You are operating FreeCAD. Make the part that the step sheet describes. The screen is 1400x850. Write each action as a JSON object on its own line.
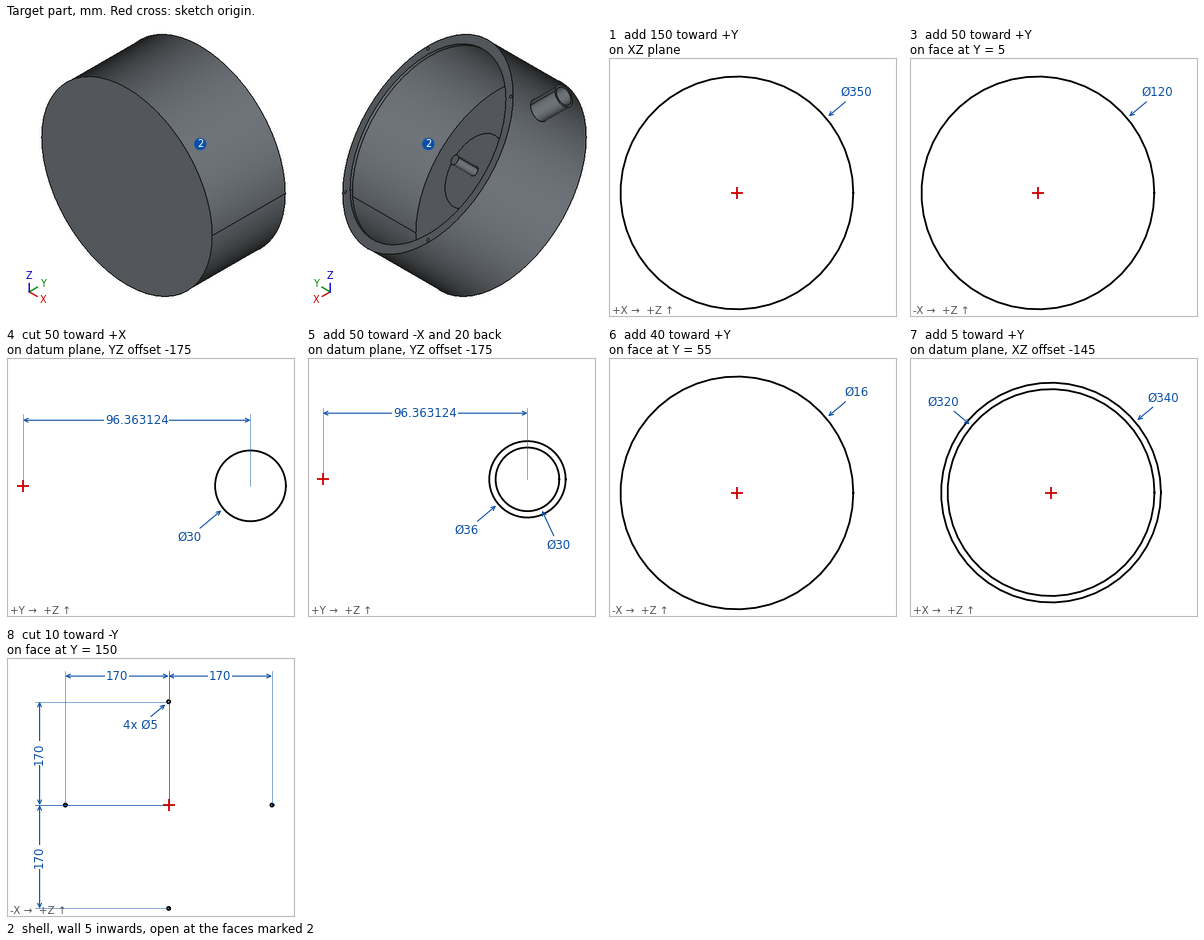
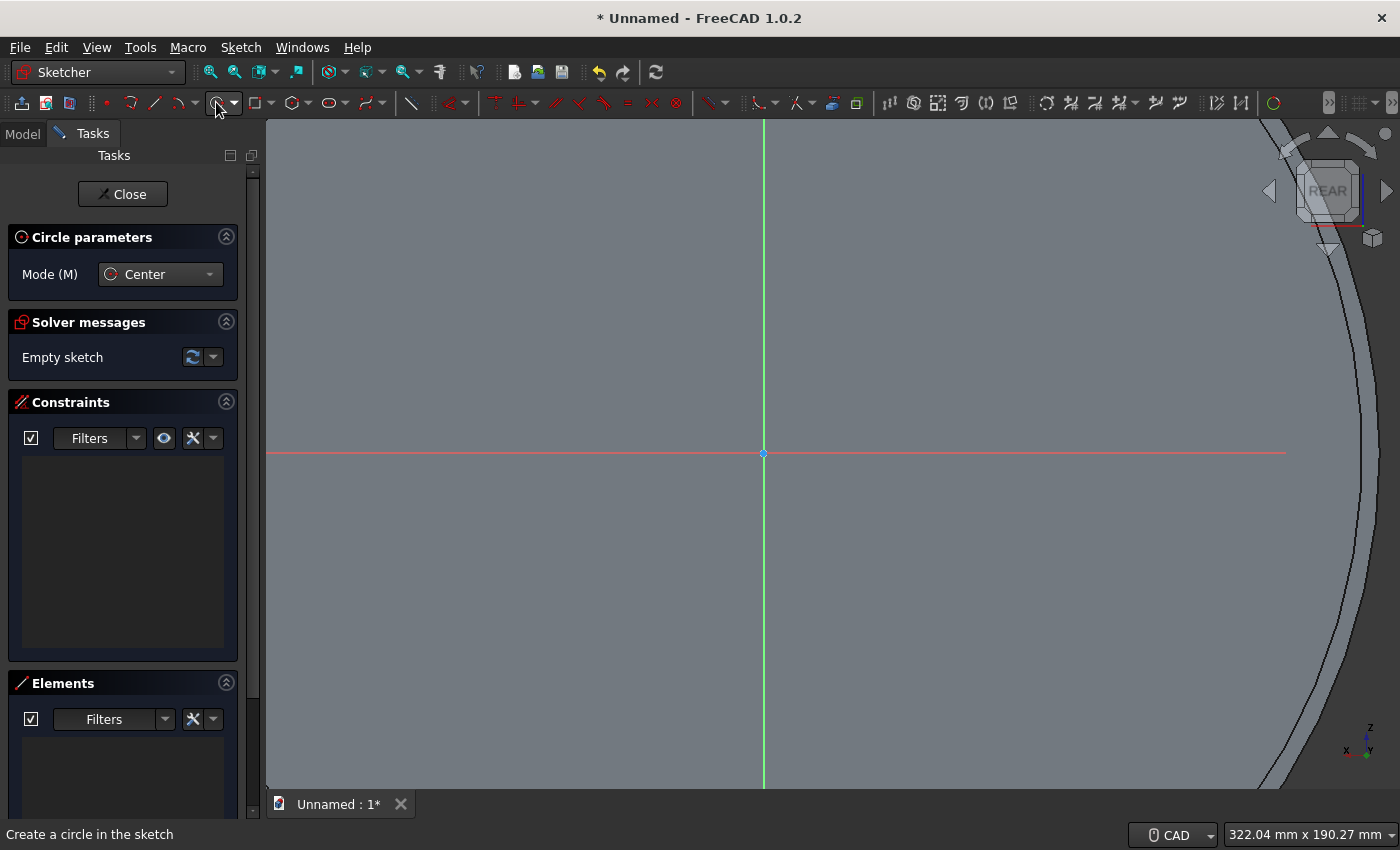
{"action": "left_click", "coordinate": [764, 453]}
{"action": "mouse_move", "coordinate": [913, 304]}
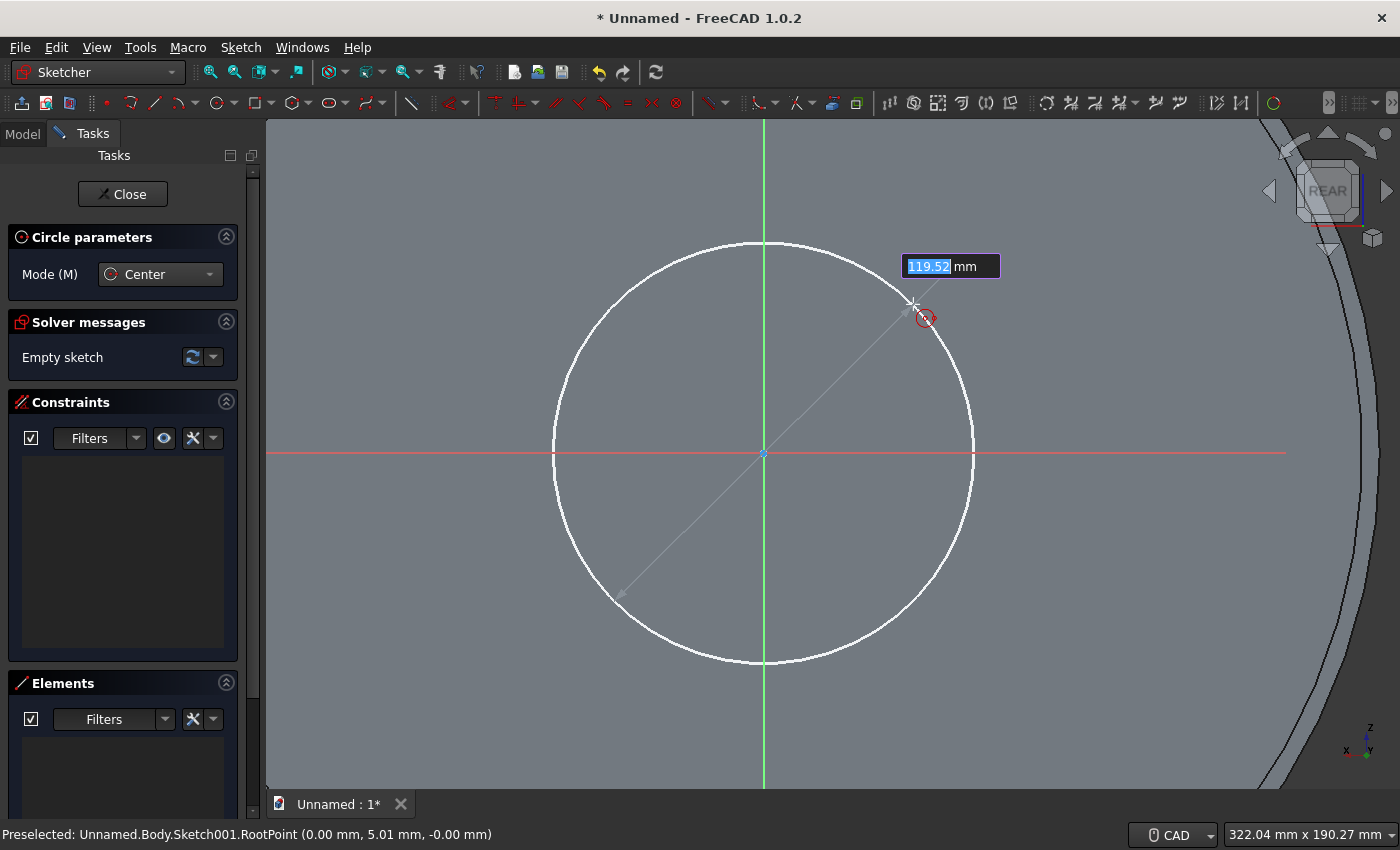
{"action": "type", "text": "120"}
{"action": "key", "text": "Return"}
{"action": "key", "text": "Escape"}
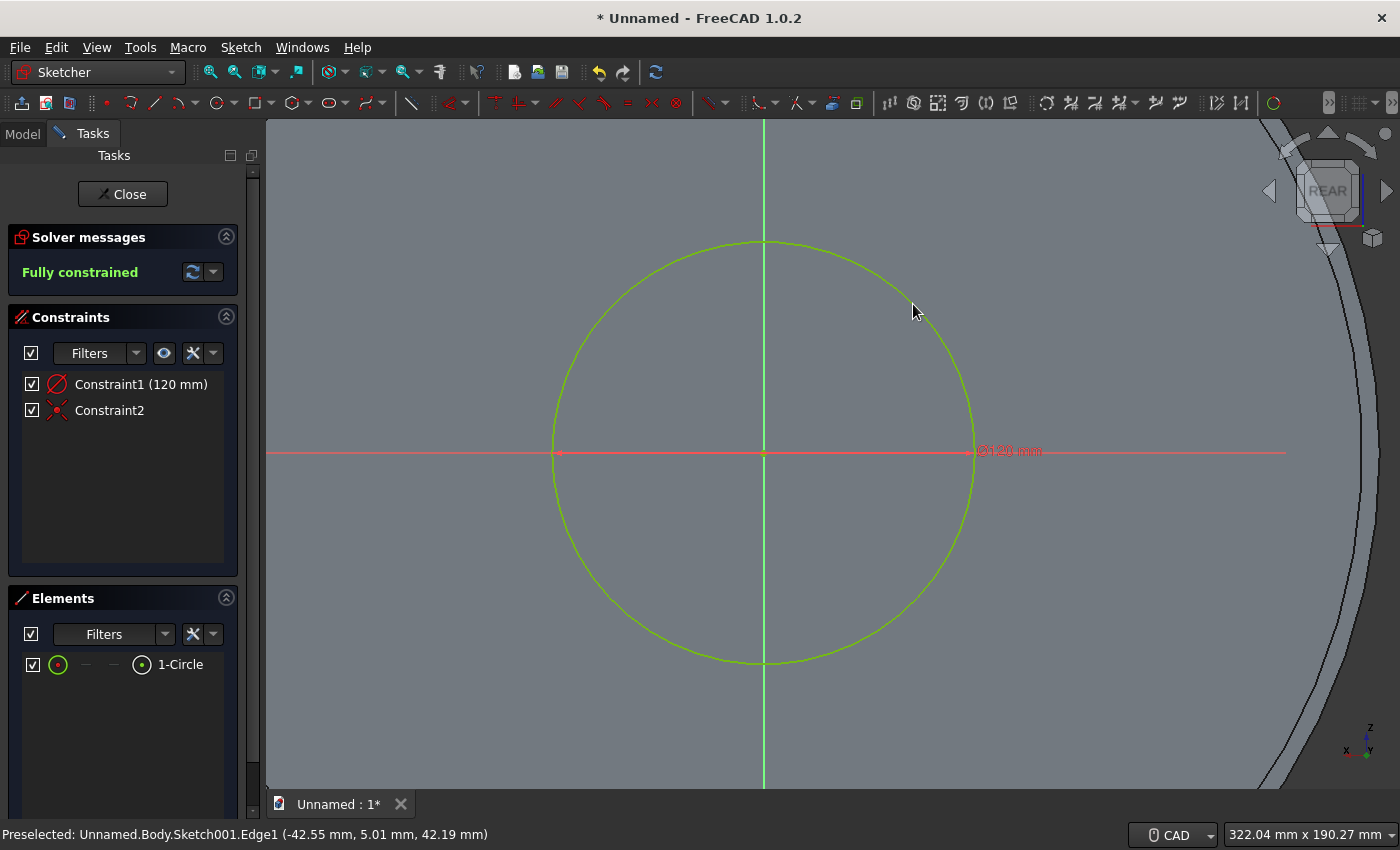
{"action": "left_click", "coordinate": [123, 194]}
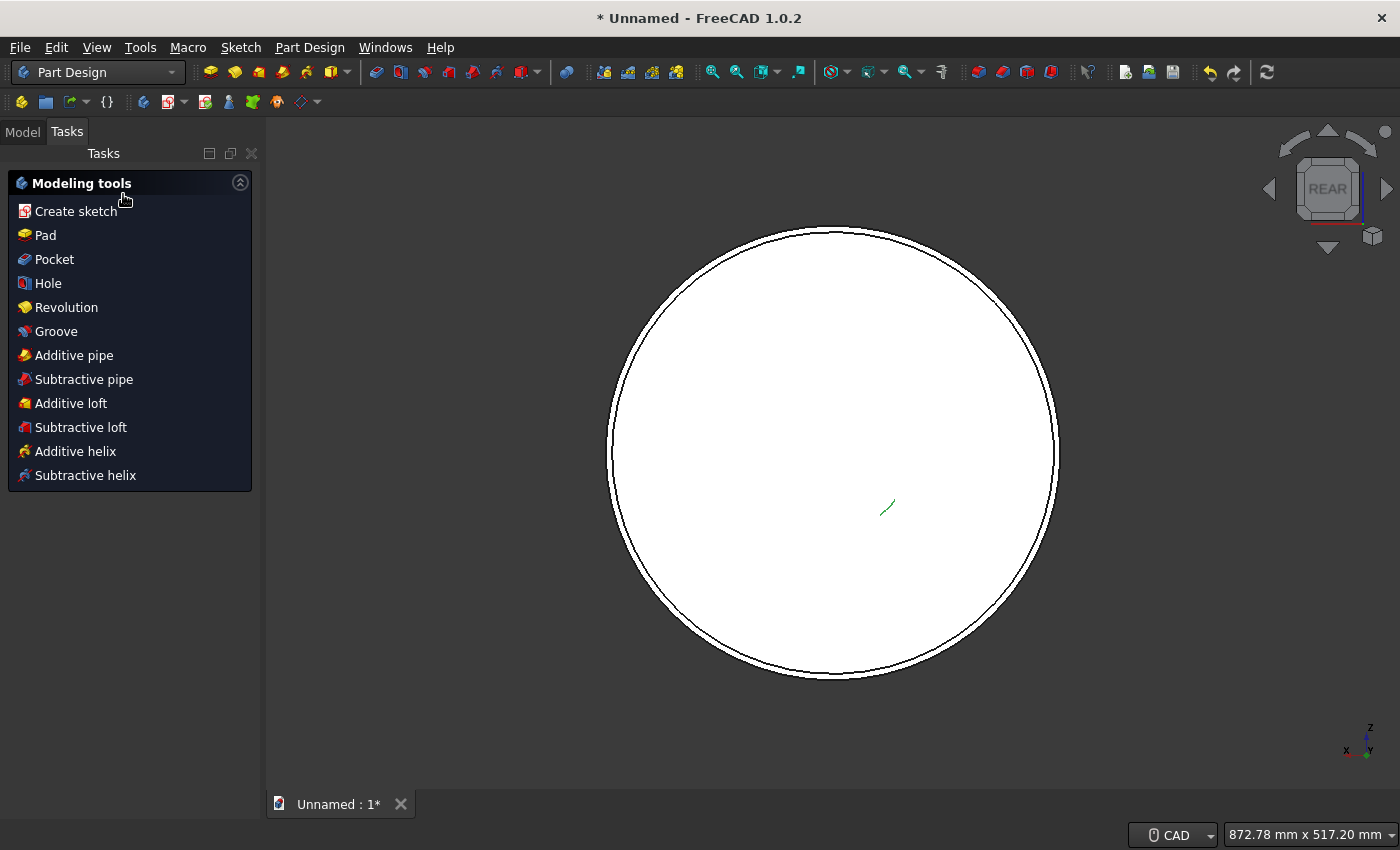
{"action": "left_click", "coordinate": [212, 72]}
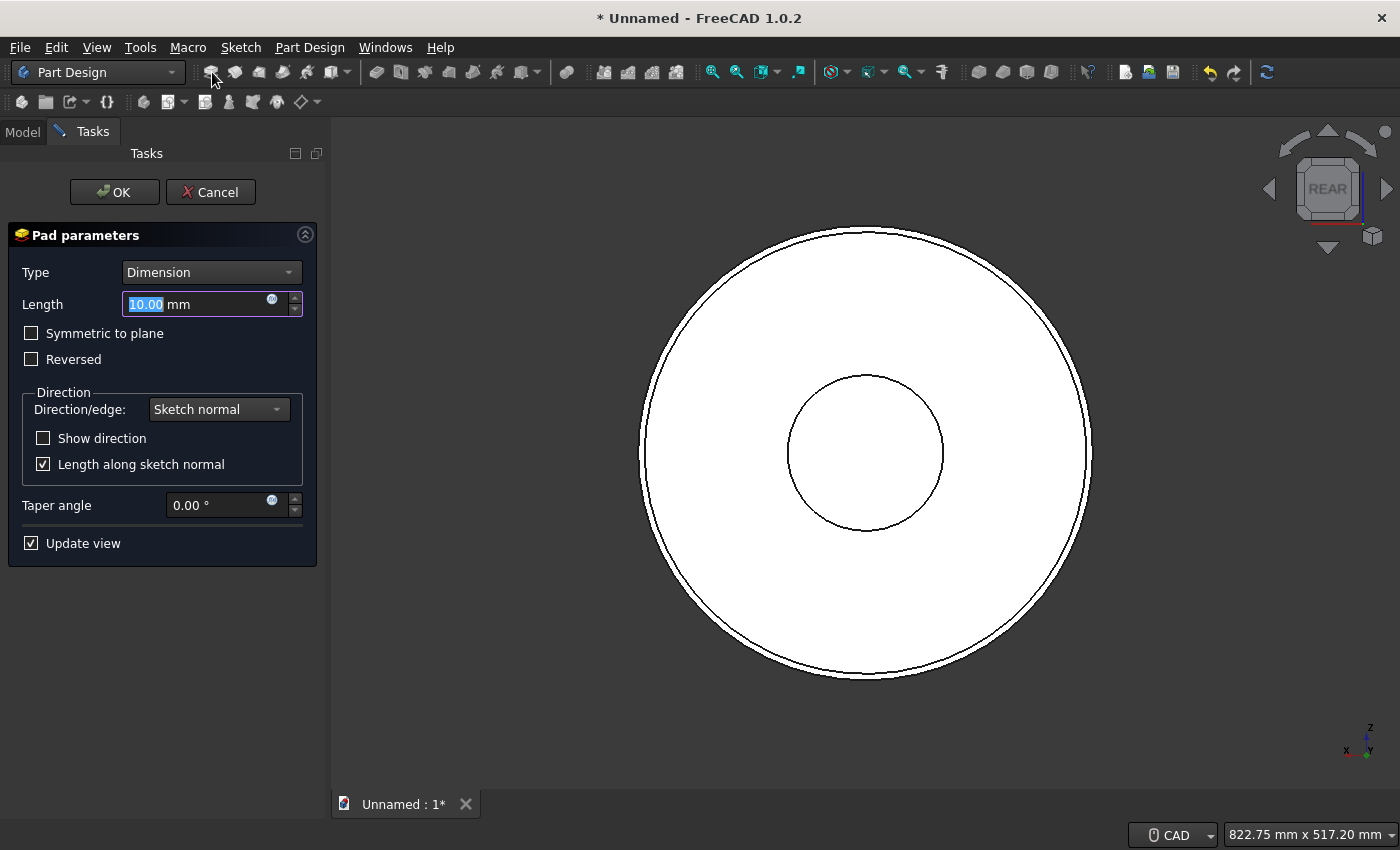
{"action": "type", "text": "50"}
{"action": "key", "text": "Tab"}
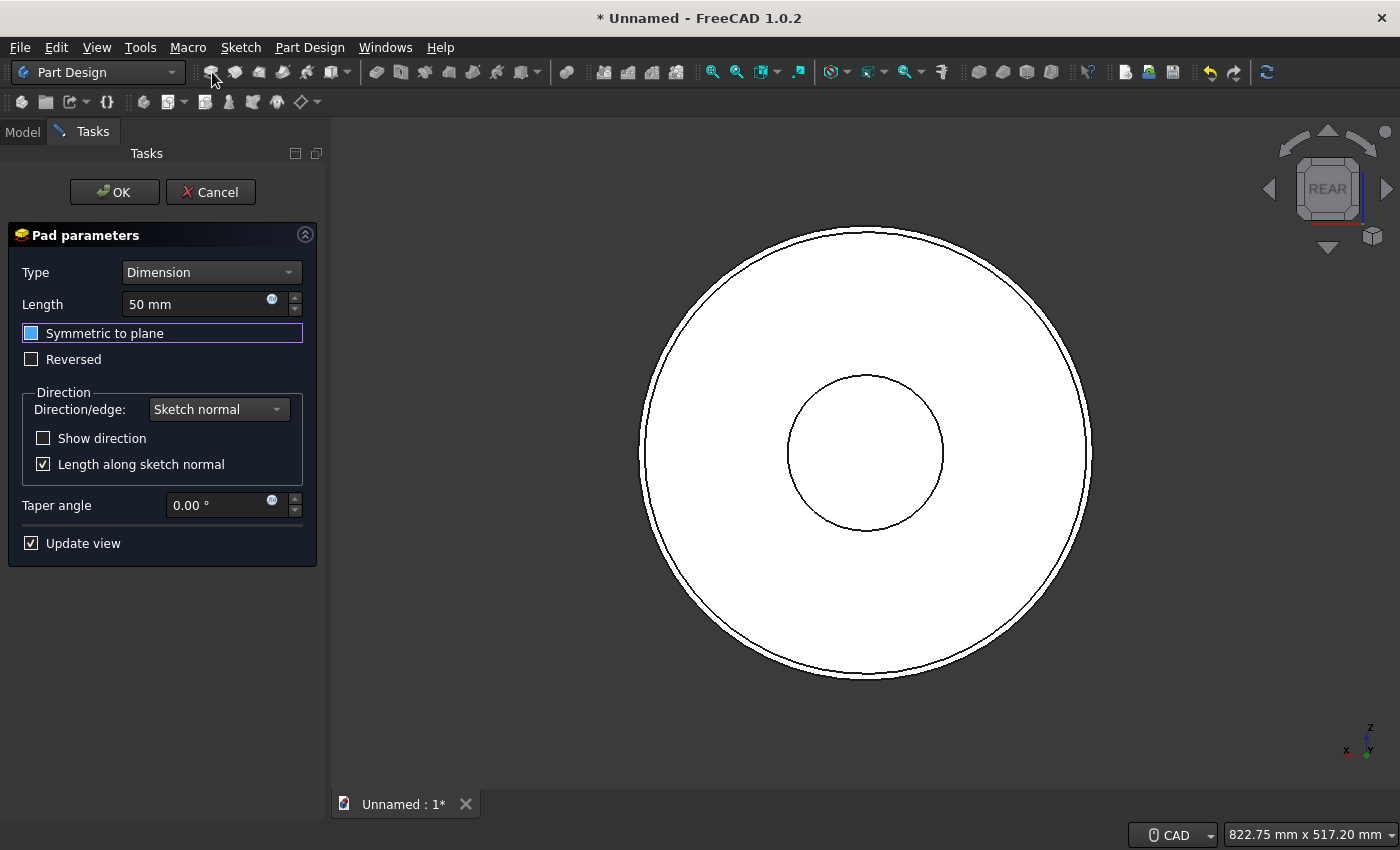
{"action": "left_click", "coordinate": [115, 192]}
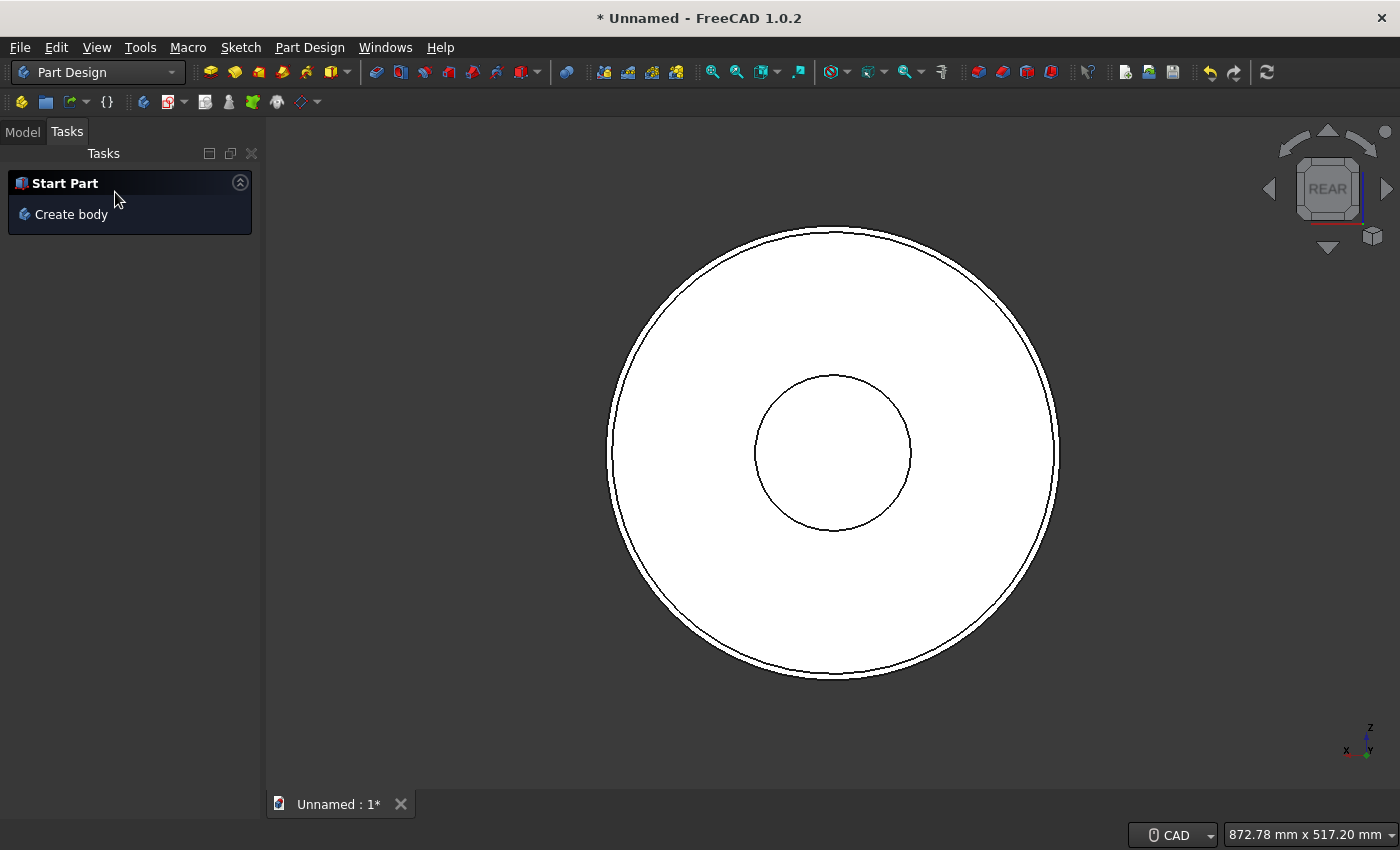
{"action": "left_click", "coordinate": [23, 131]}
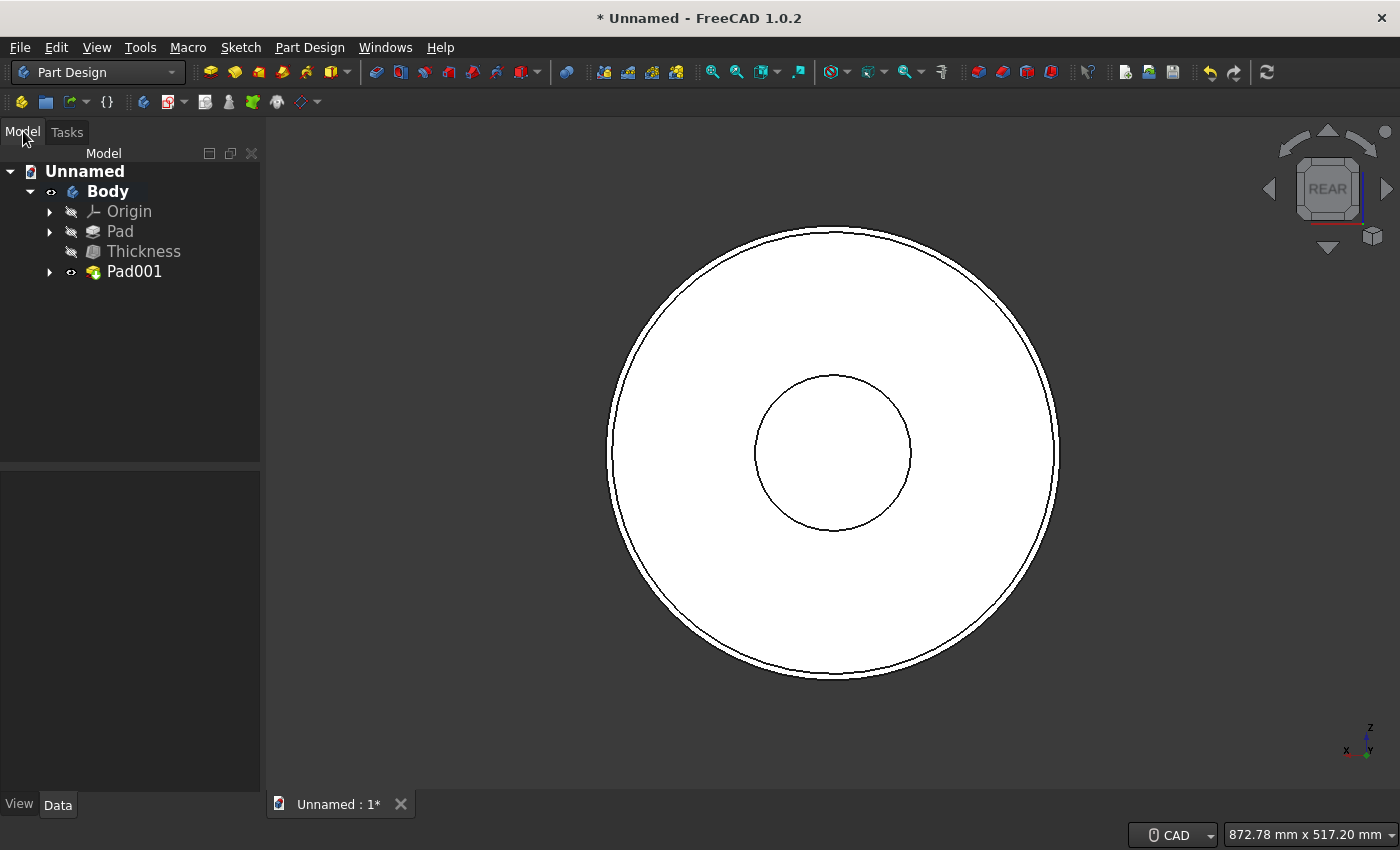
{"action": "left_click", "coordinate": [50, 212]}